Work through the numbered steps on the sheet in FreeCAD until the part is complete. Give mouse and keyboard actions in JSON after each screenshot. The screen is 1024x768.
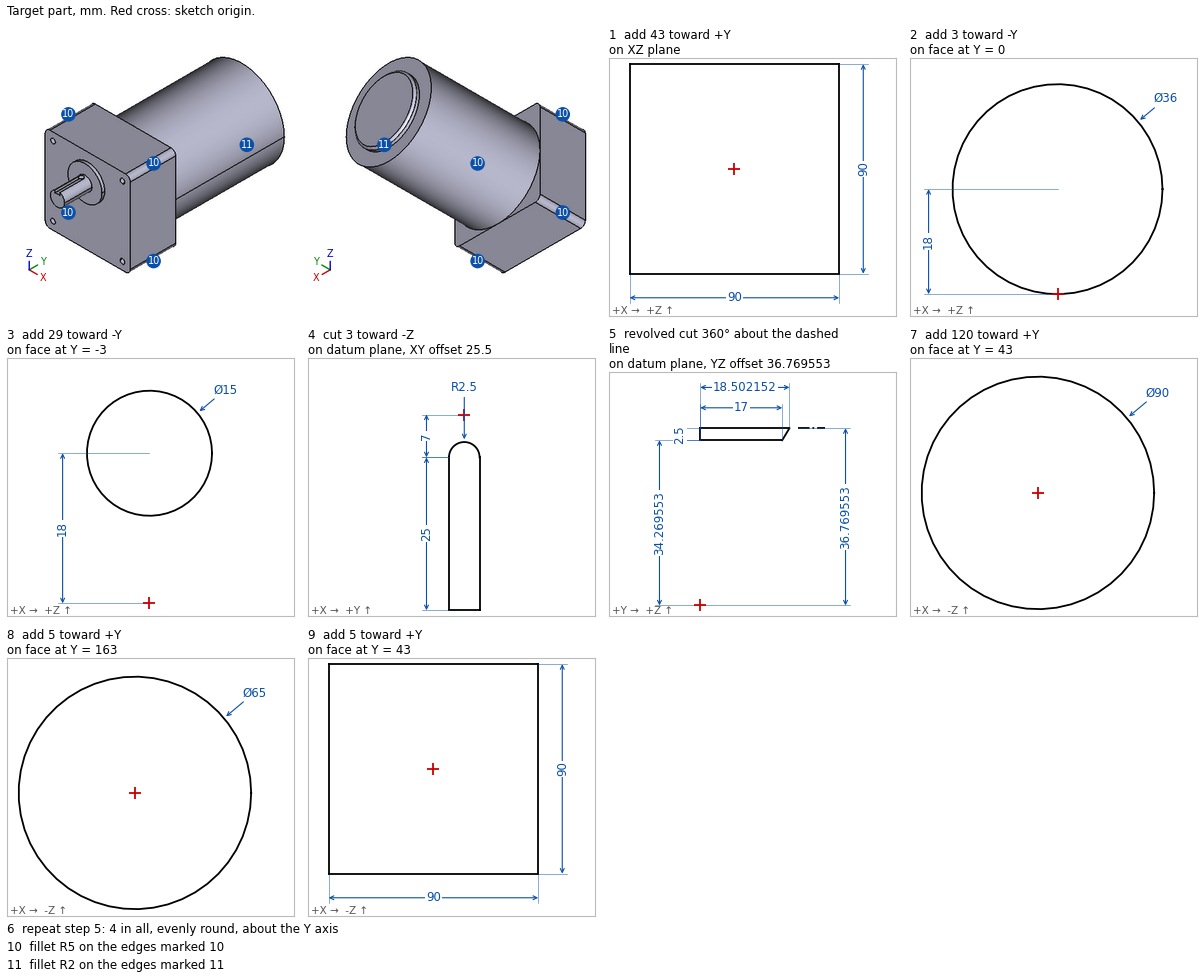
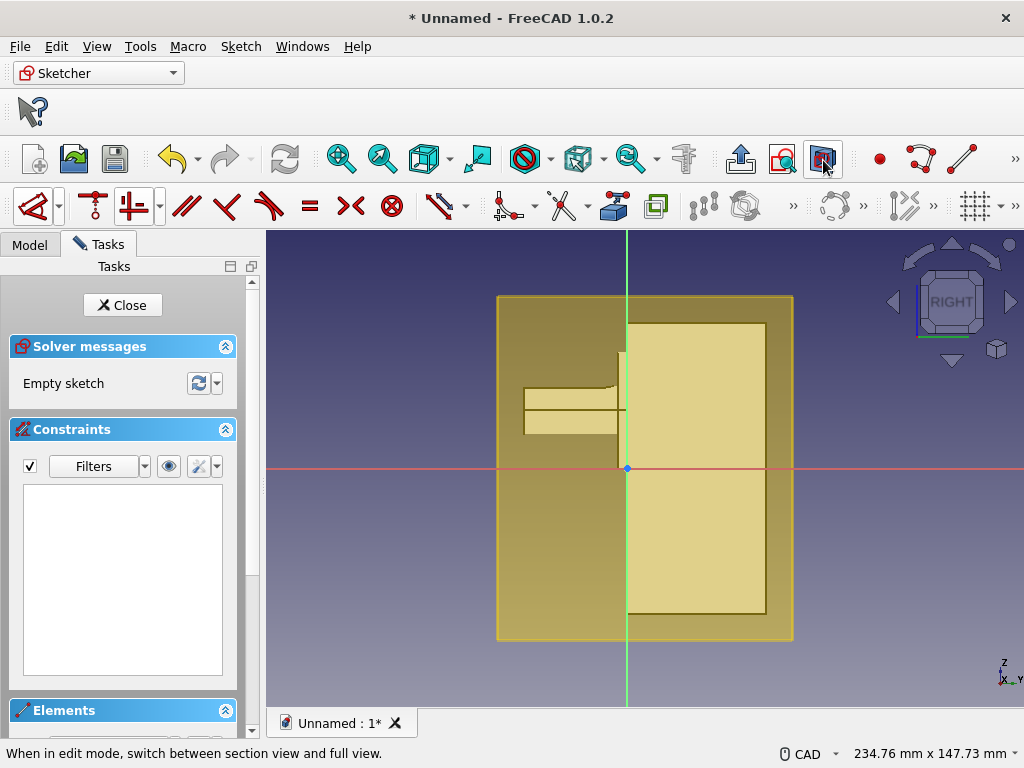
{"action": "scroll", "coordinate": [723, 375], "scroll_direction": "up", "scroll_amount": 5}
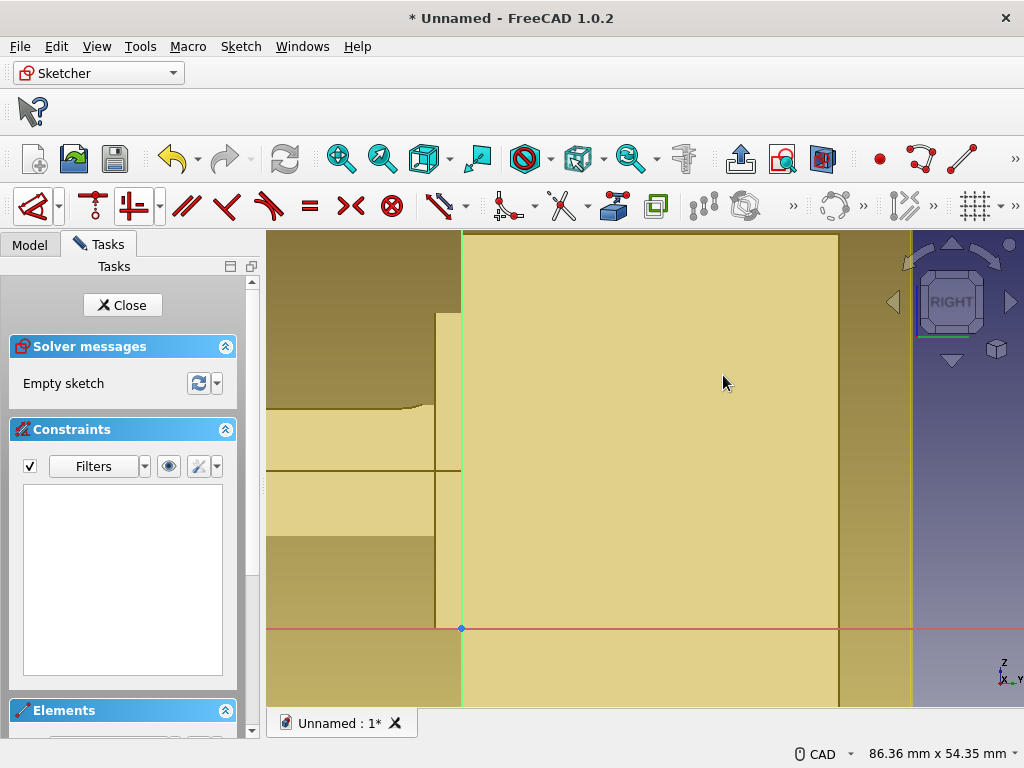
{"action": "left_click", "coordinate": [921, 160]}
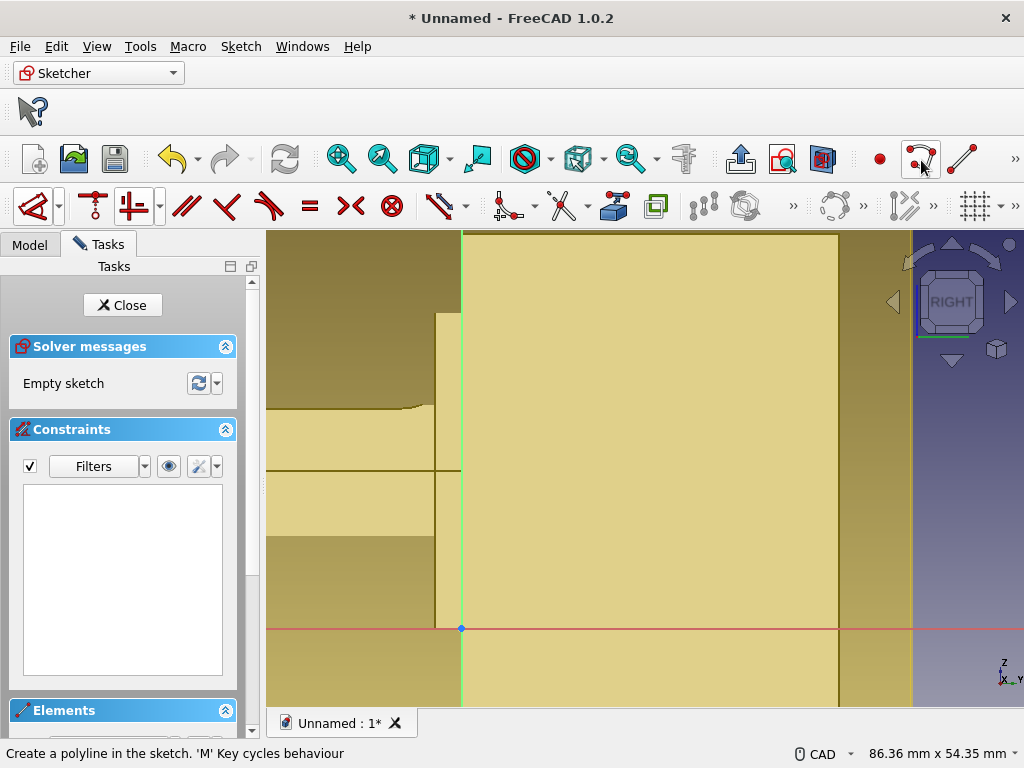
{"action": "left_click", "coordinate": [462, 328]}
{"action": "left_click", "coordinate": [611, 328]}
{"action": "left_click", "coordinate": [624, 306]}
{"action": "left_click", "coordinate": [471, 306]}
{"action": "left_click", "coordinate": [462, 329]}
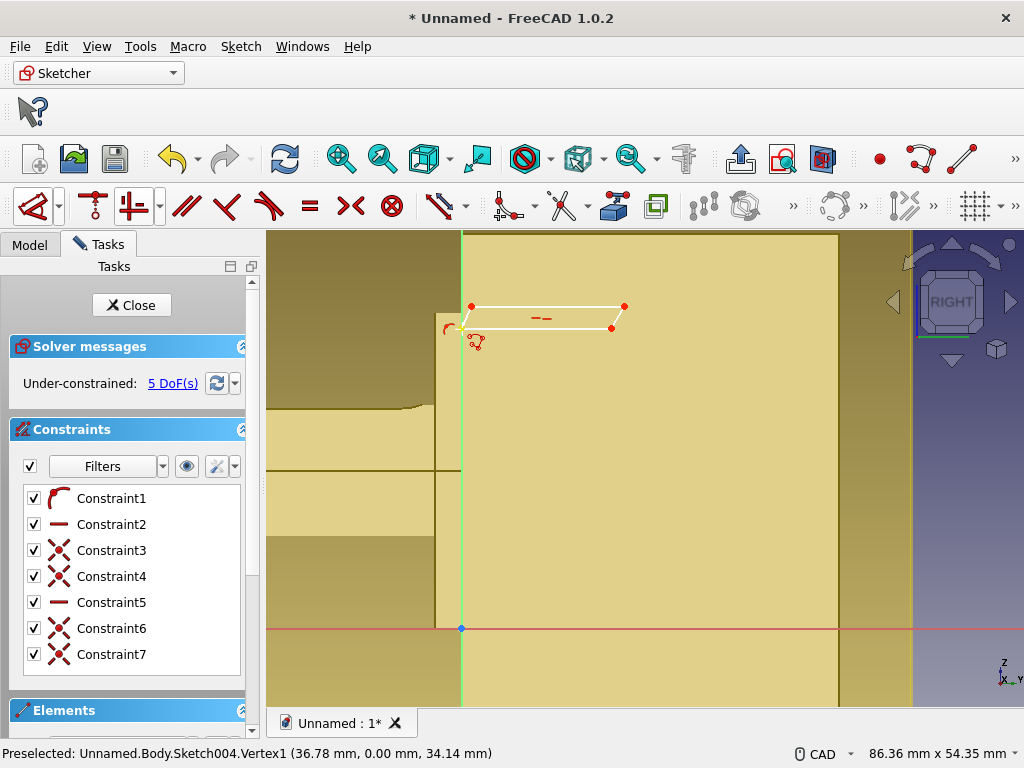
{"action": "left_click", "coordinate": [962, 160]}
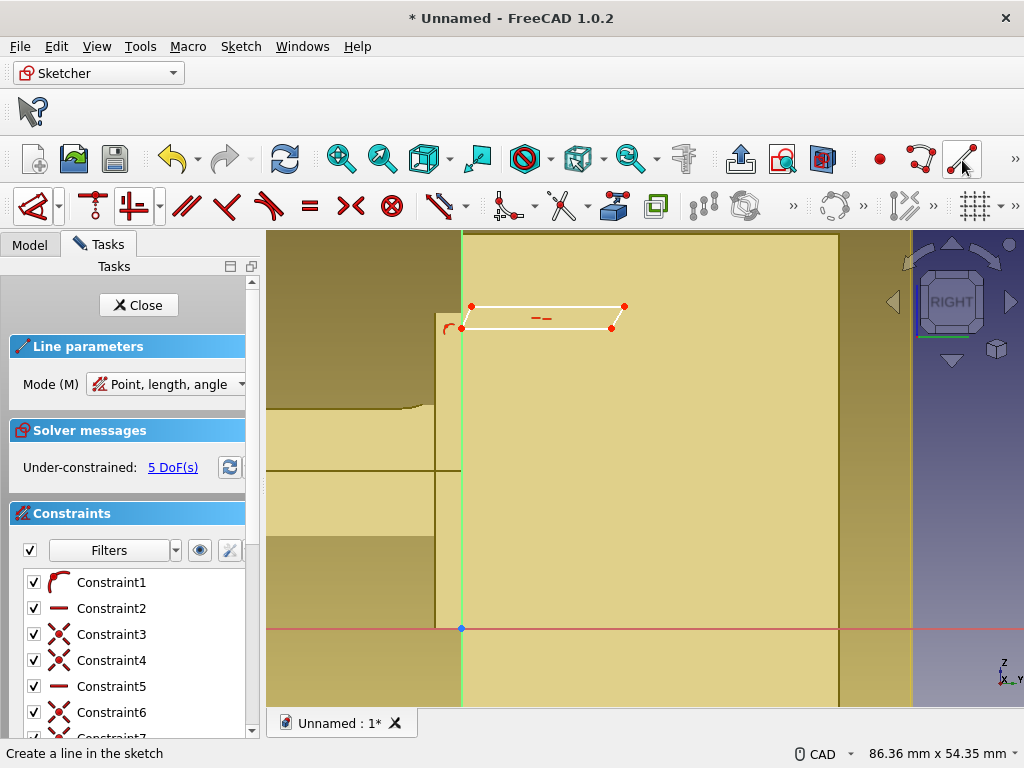
{"action": "left_click", "coordinate": [640, 306]}
{"action": "left_click", "coordinate": [689, 306]}
{"action": "key", "text": "Escape"}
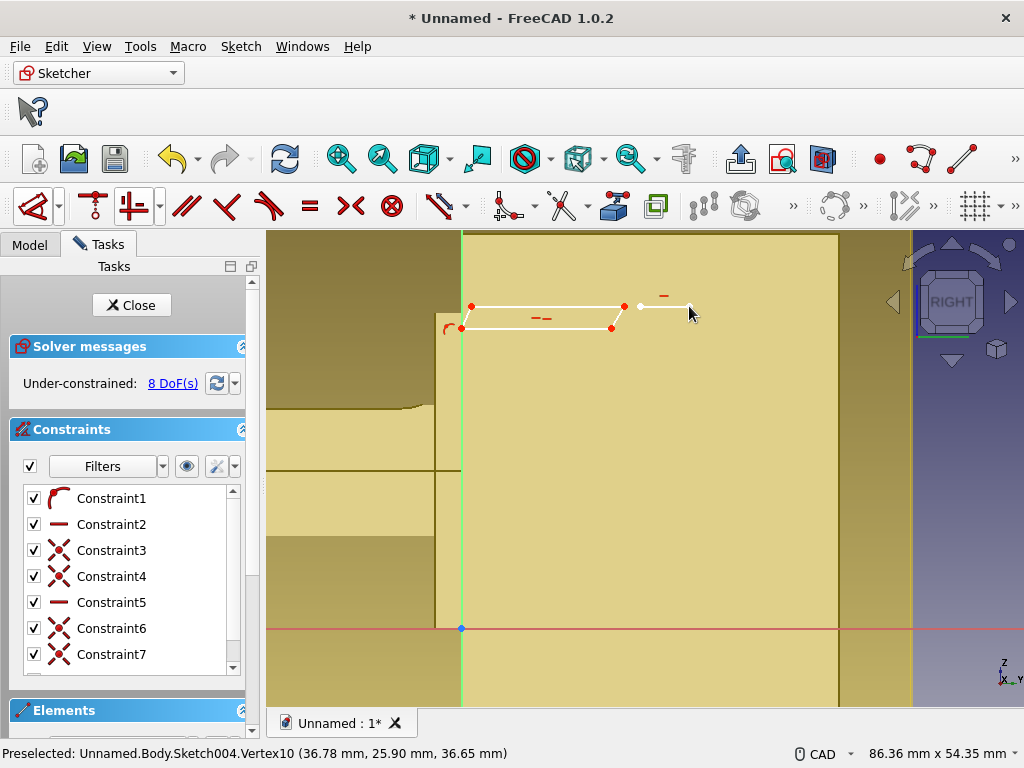
{"action": "left_click", "coordinate": [655, 307]}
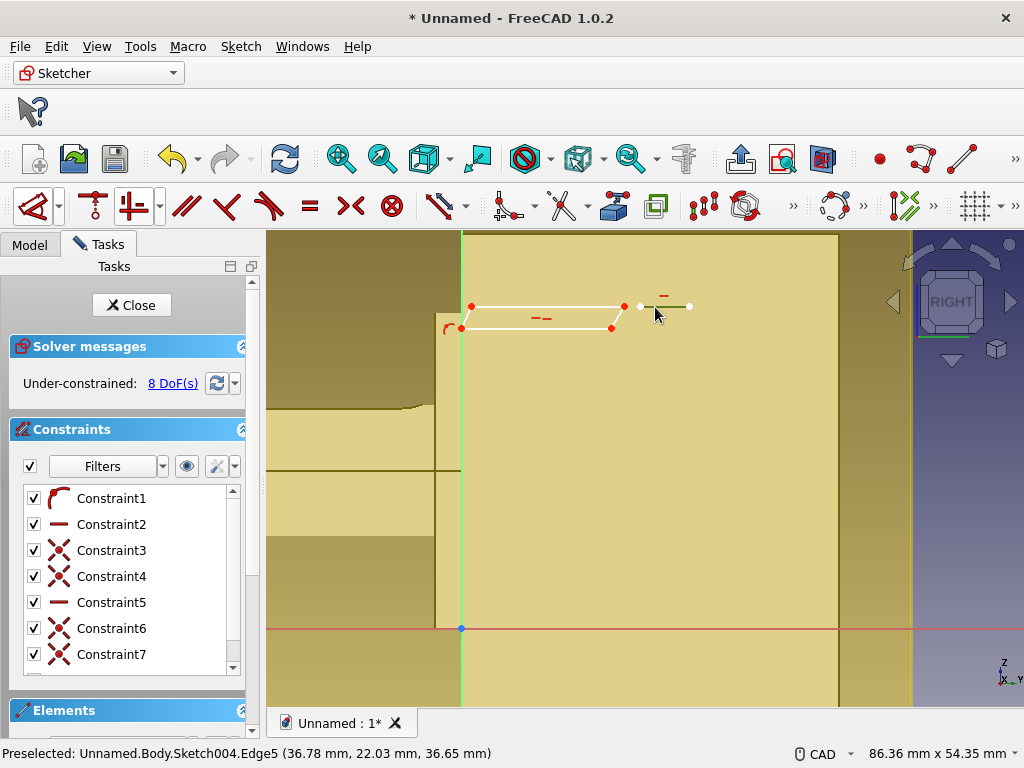
{"action": "key", "text": "g n"}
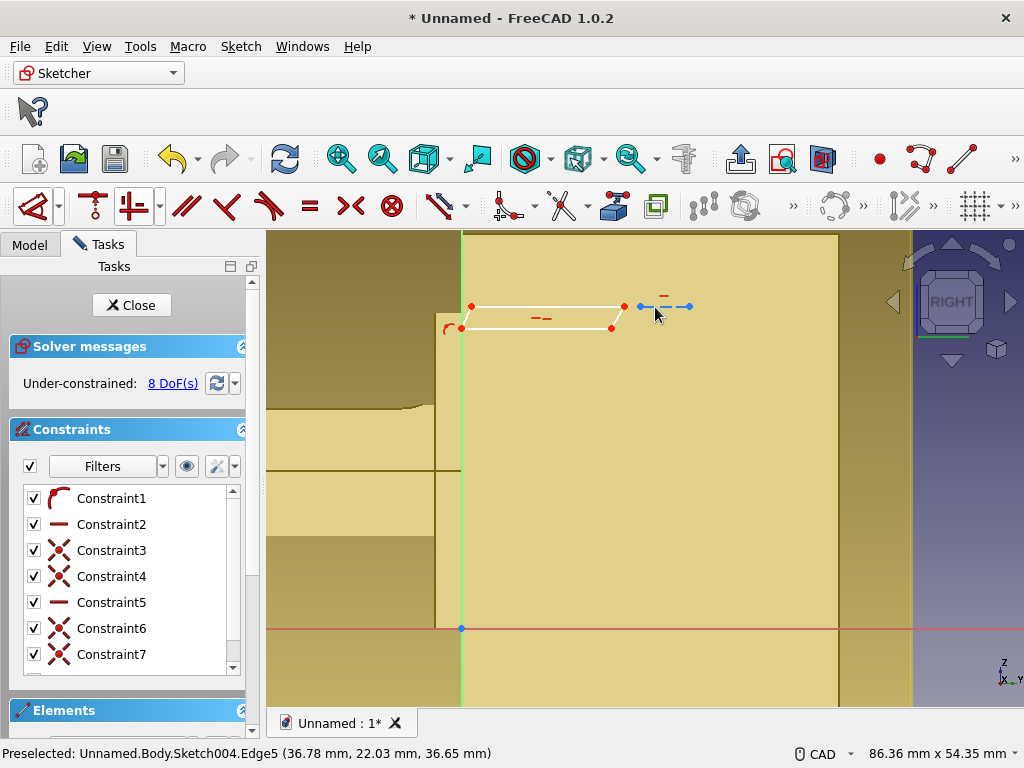
{"action": "scroll", "coordinate": [465, 320], "scroll_direction": "up", "scroll_amount": 3}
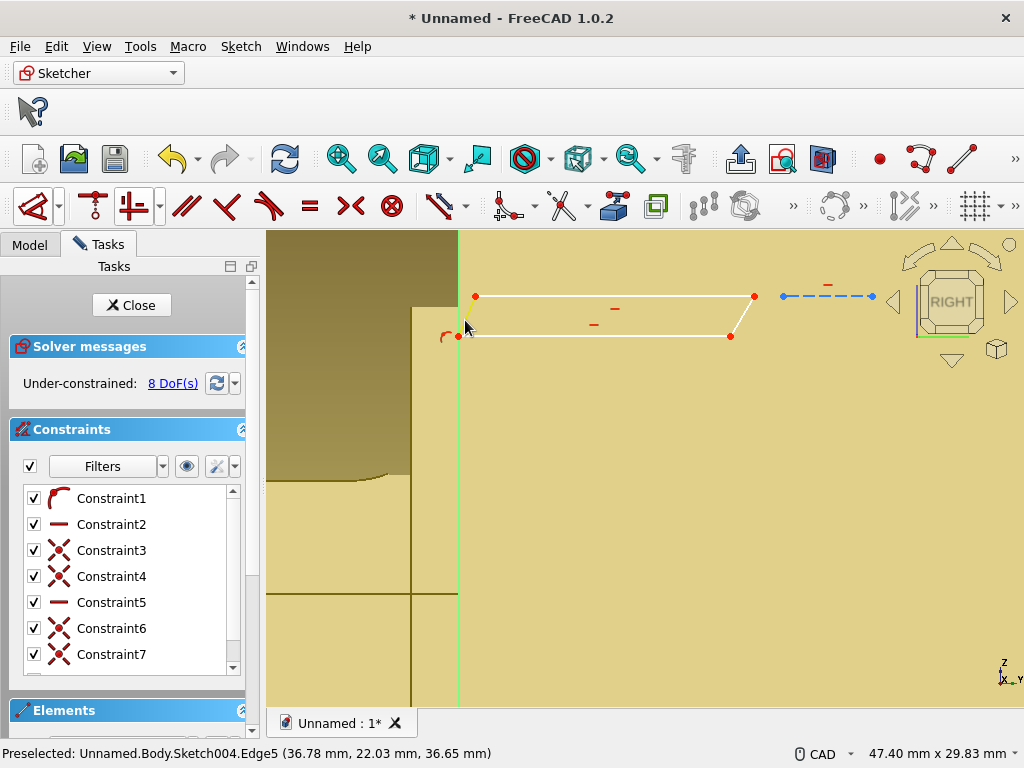
{"action": "left_click", "coordinate": [466, 320]}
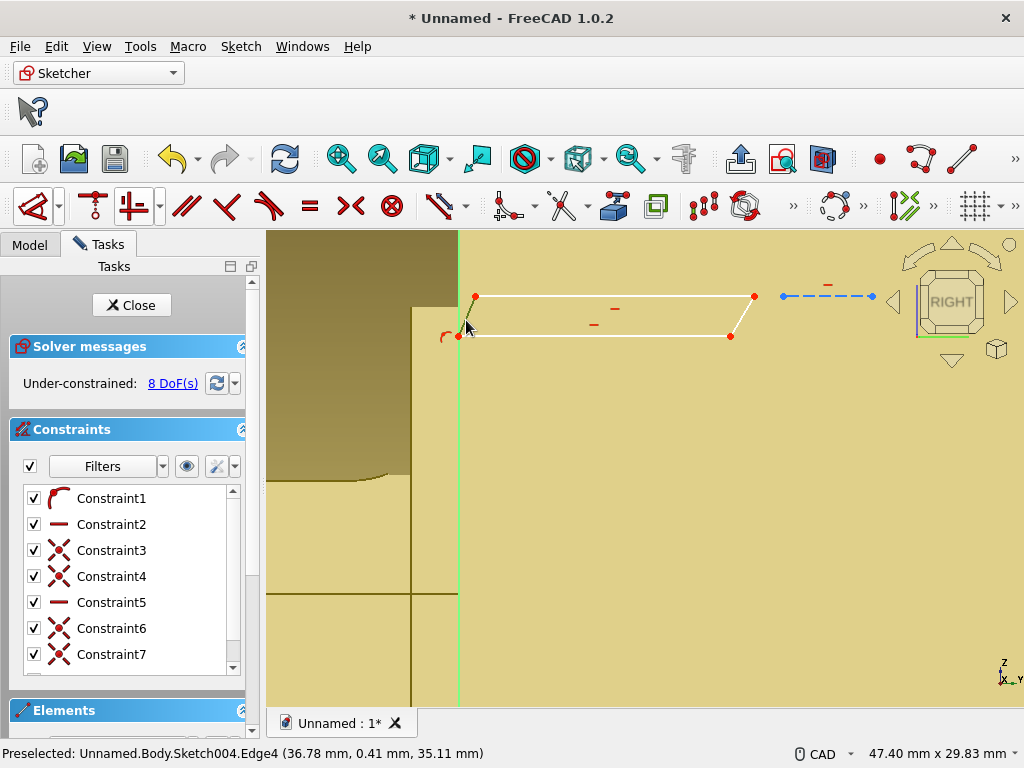
{"action": "left_click", "coordinate": [160, 206]}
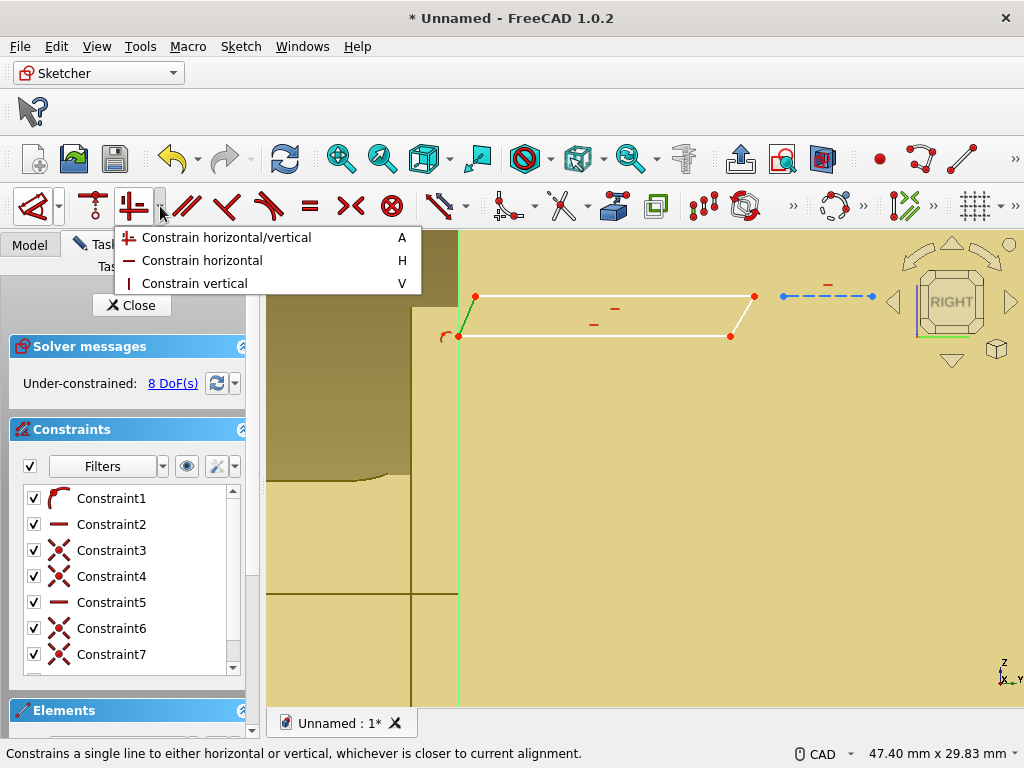
{"action": "left_click", "coordinate": [268, 284]}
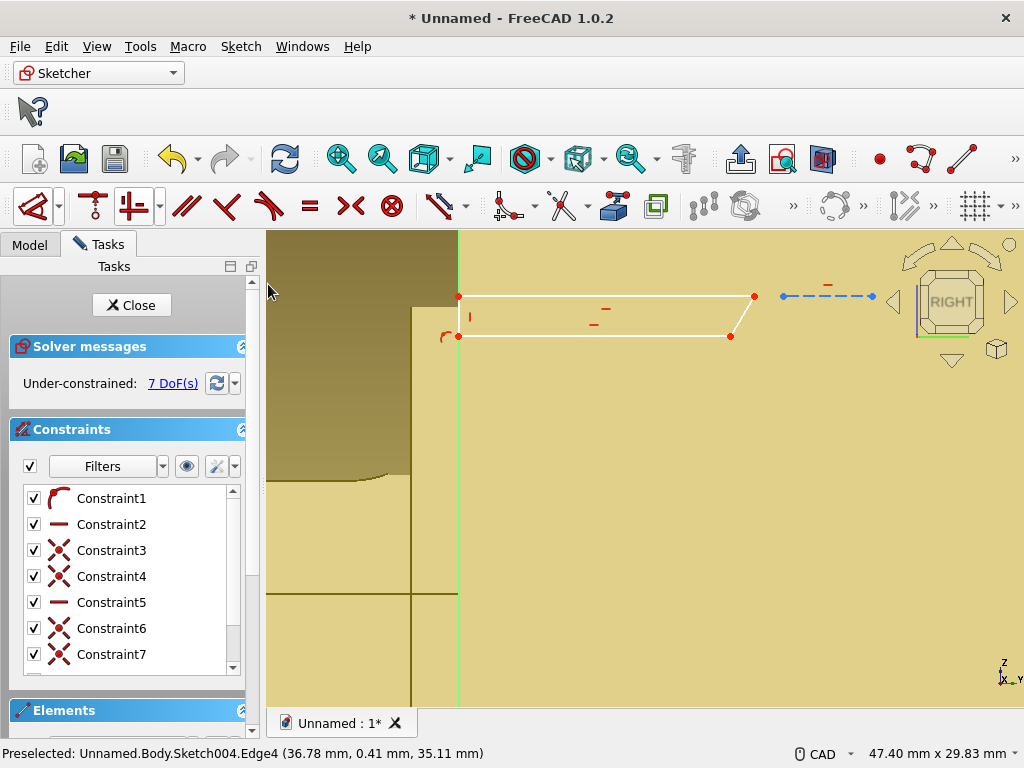
{"action": "left_click", "coordinate": [540, 336]}